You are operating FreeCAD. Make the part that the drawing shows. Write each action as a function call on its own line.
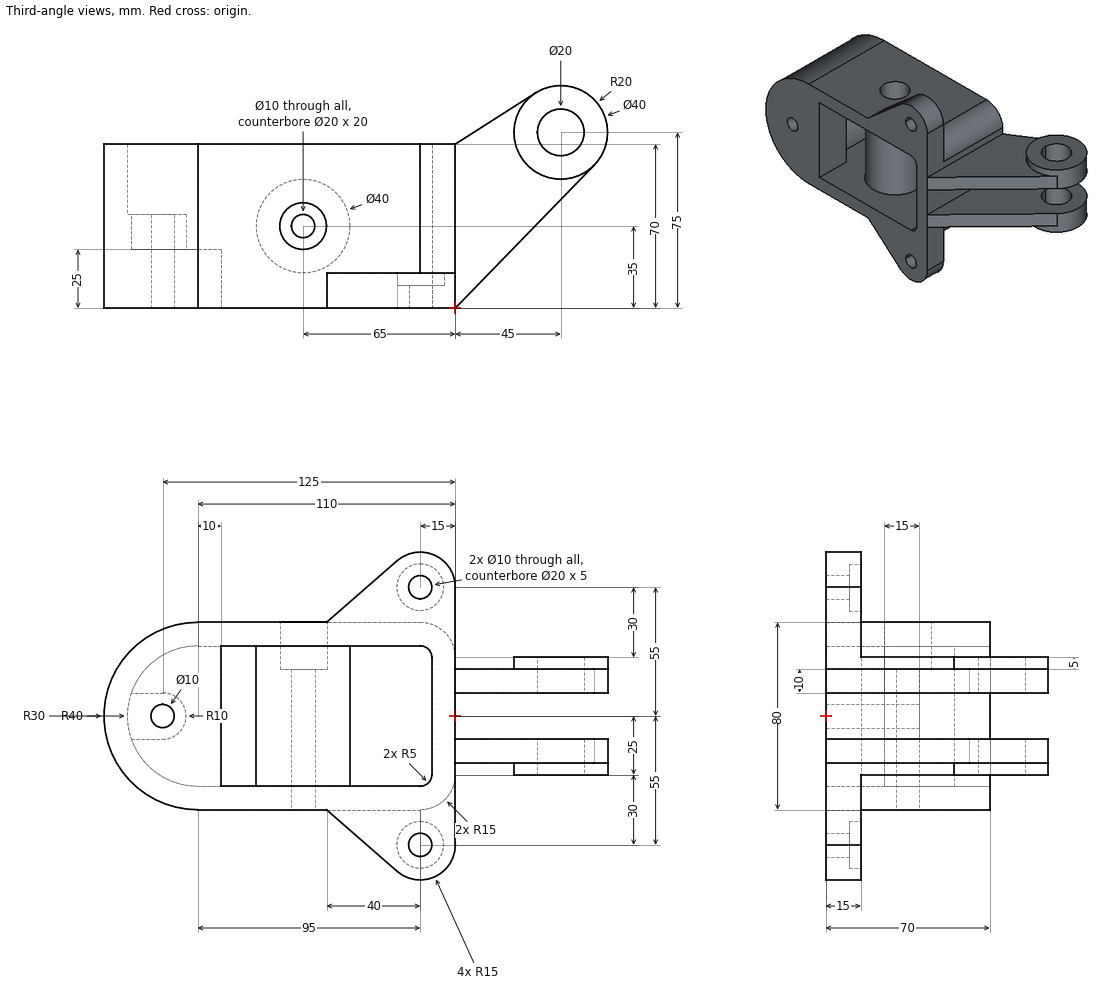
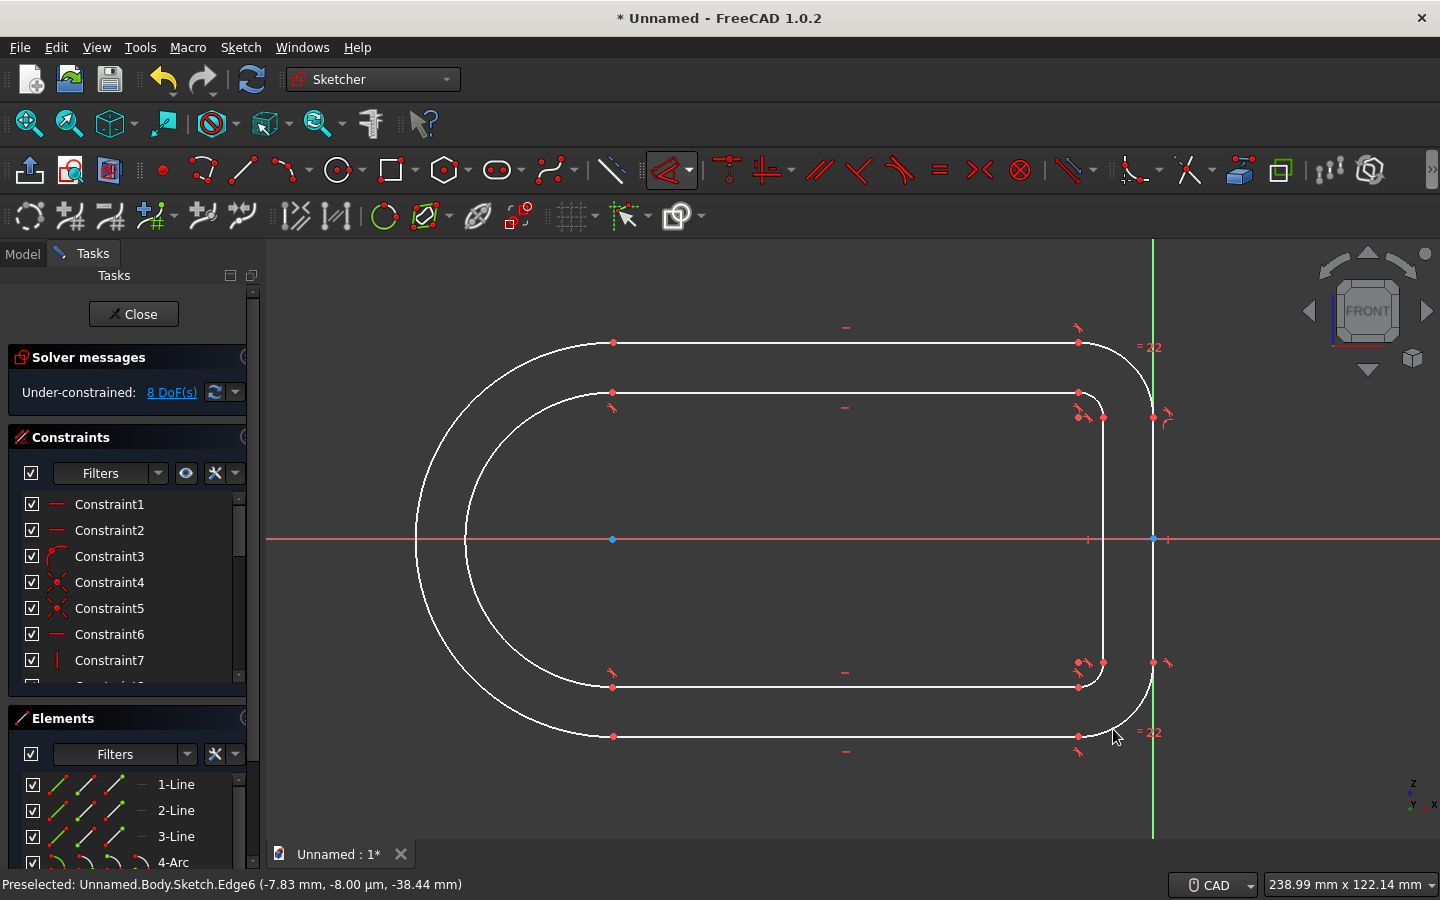
click(613, 540)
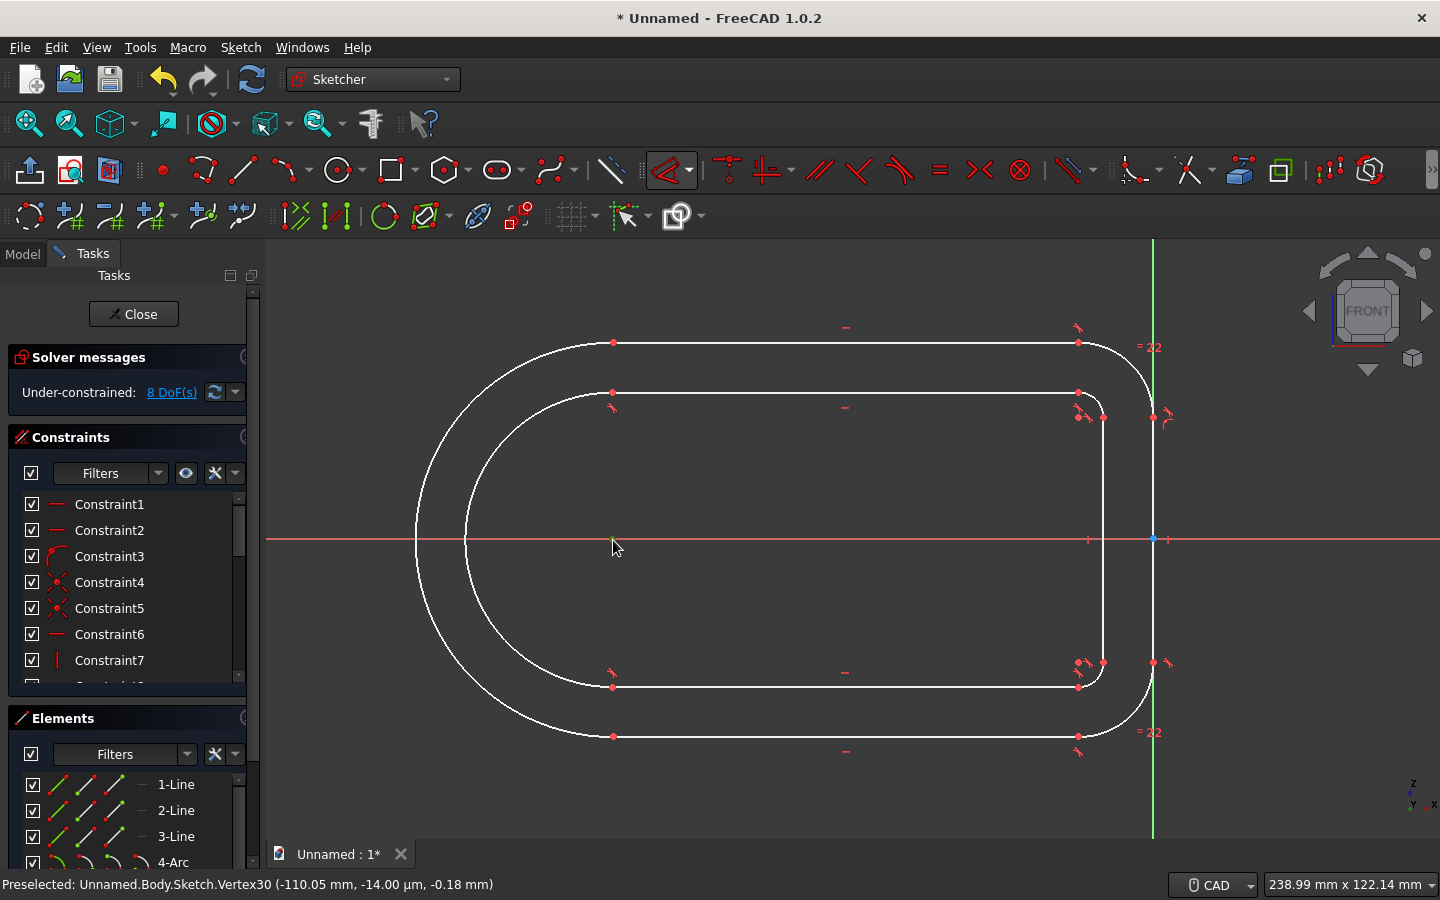
click(364, 539)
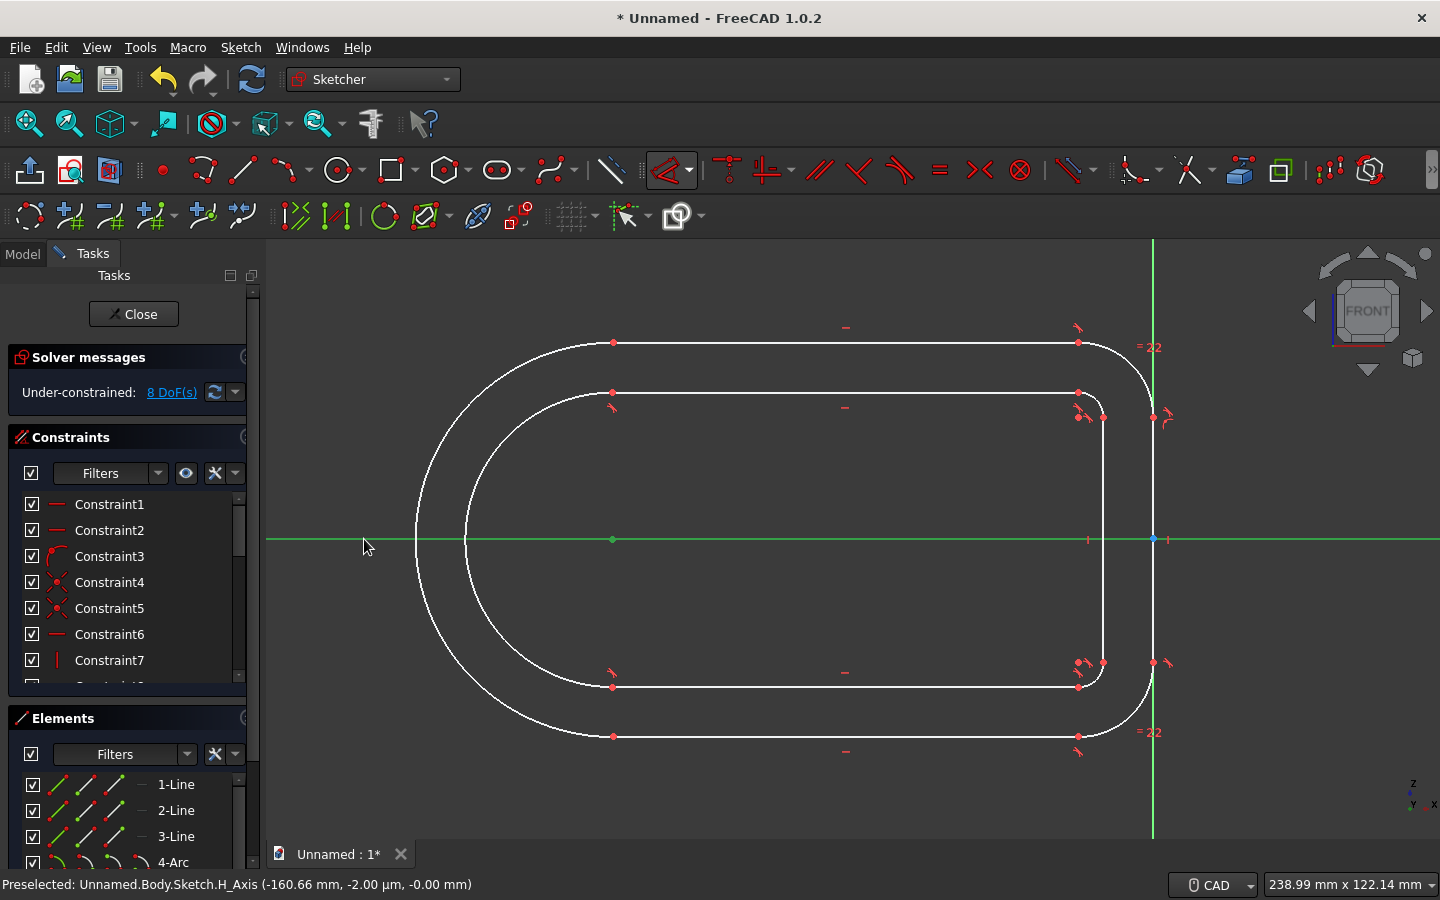
click(728, 170)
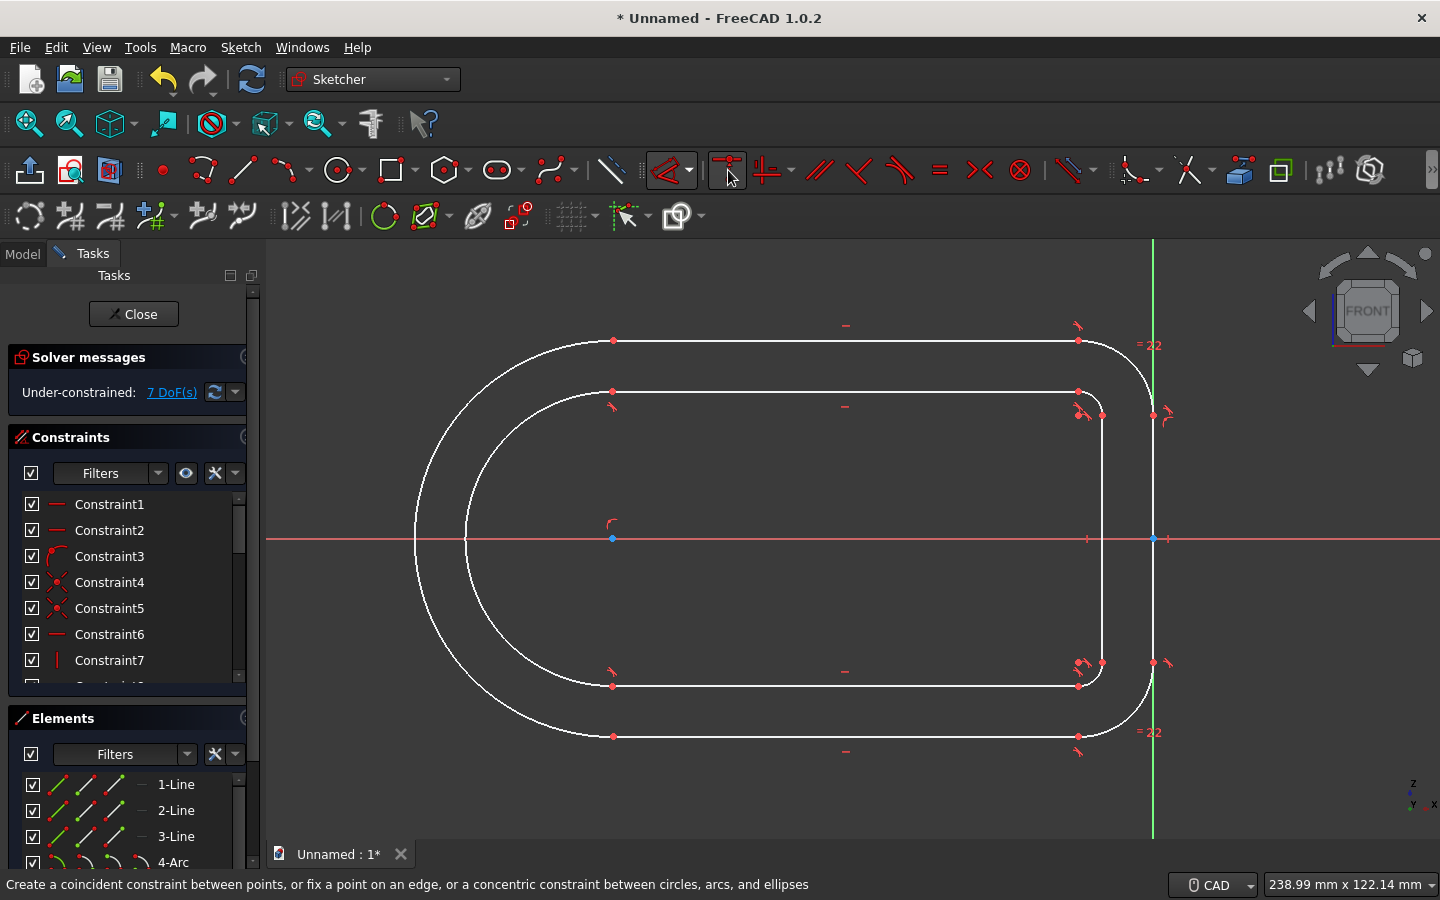
click(453, 422)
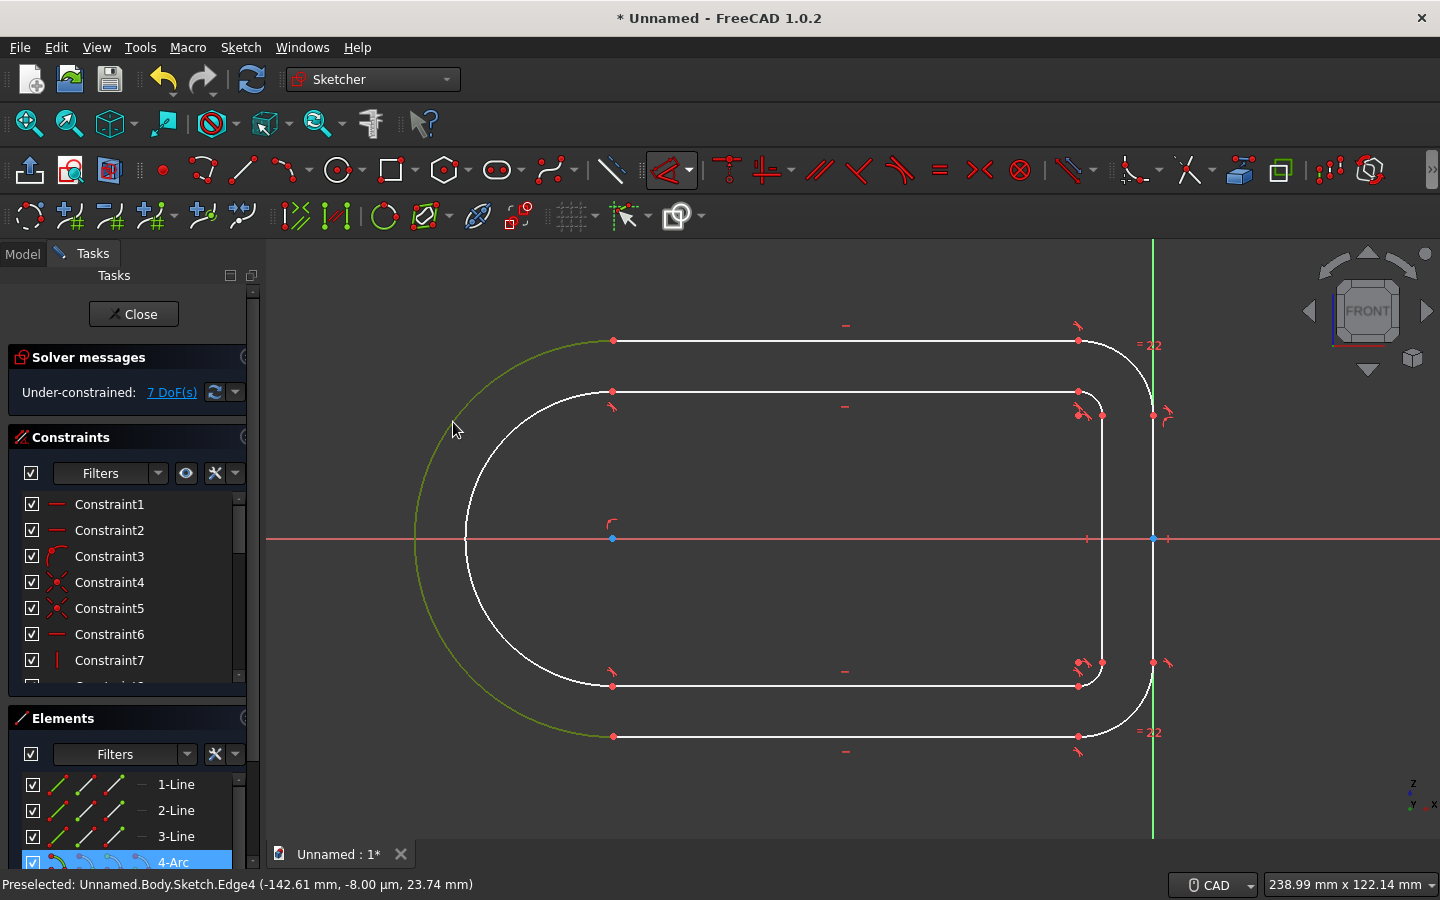
key(k)
key(r)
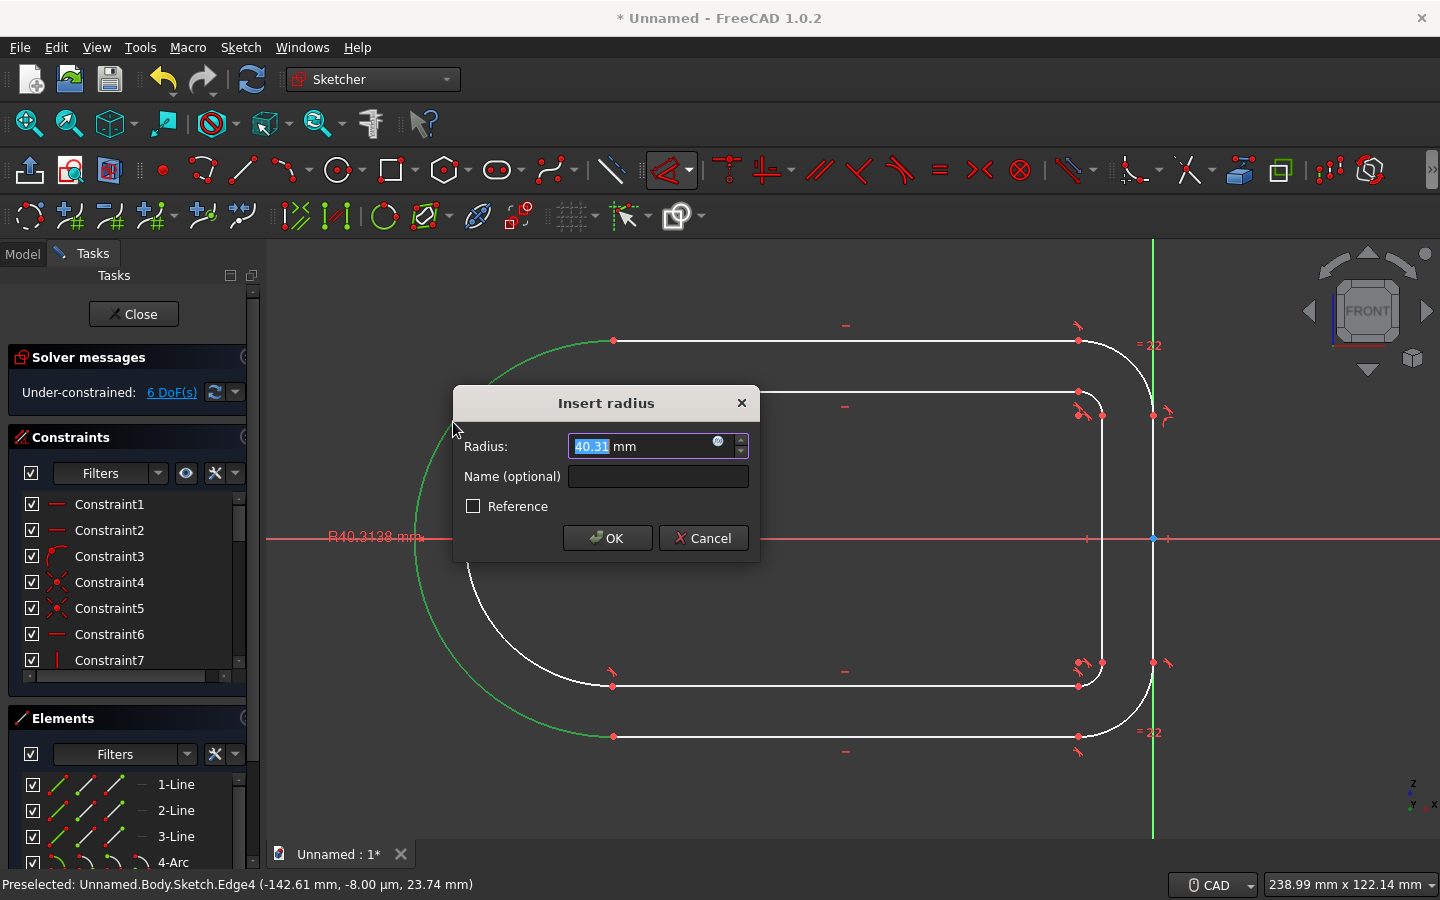
text(40)
key(Return)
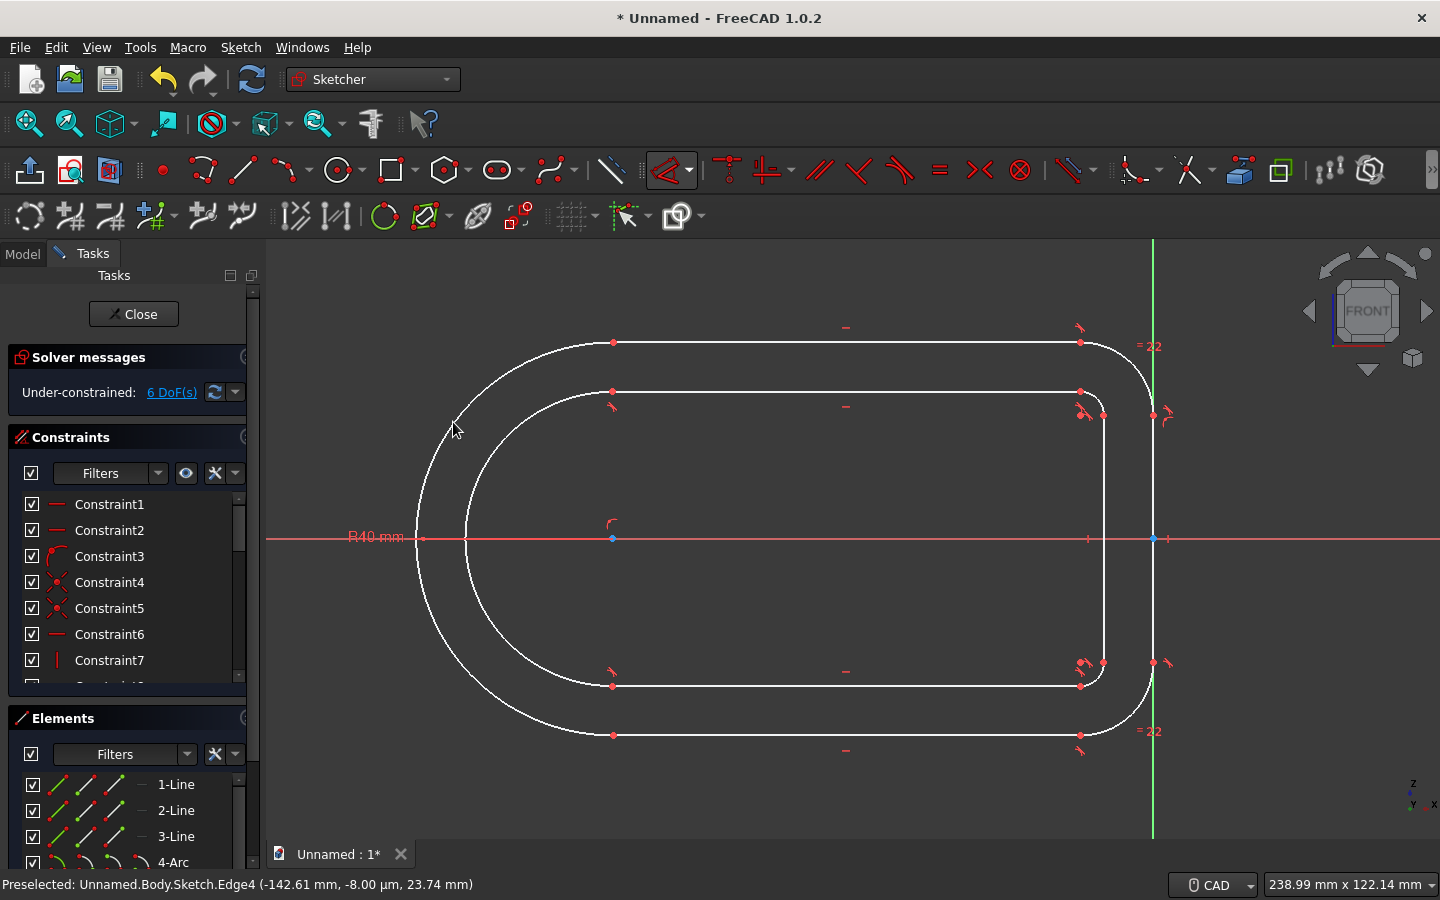
click(1114, 350)